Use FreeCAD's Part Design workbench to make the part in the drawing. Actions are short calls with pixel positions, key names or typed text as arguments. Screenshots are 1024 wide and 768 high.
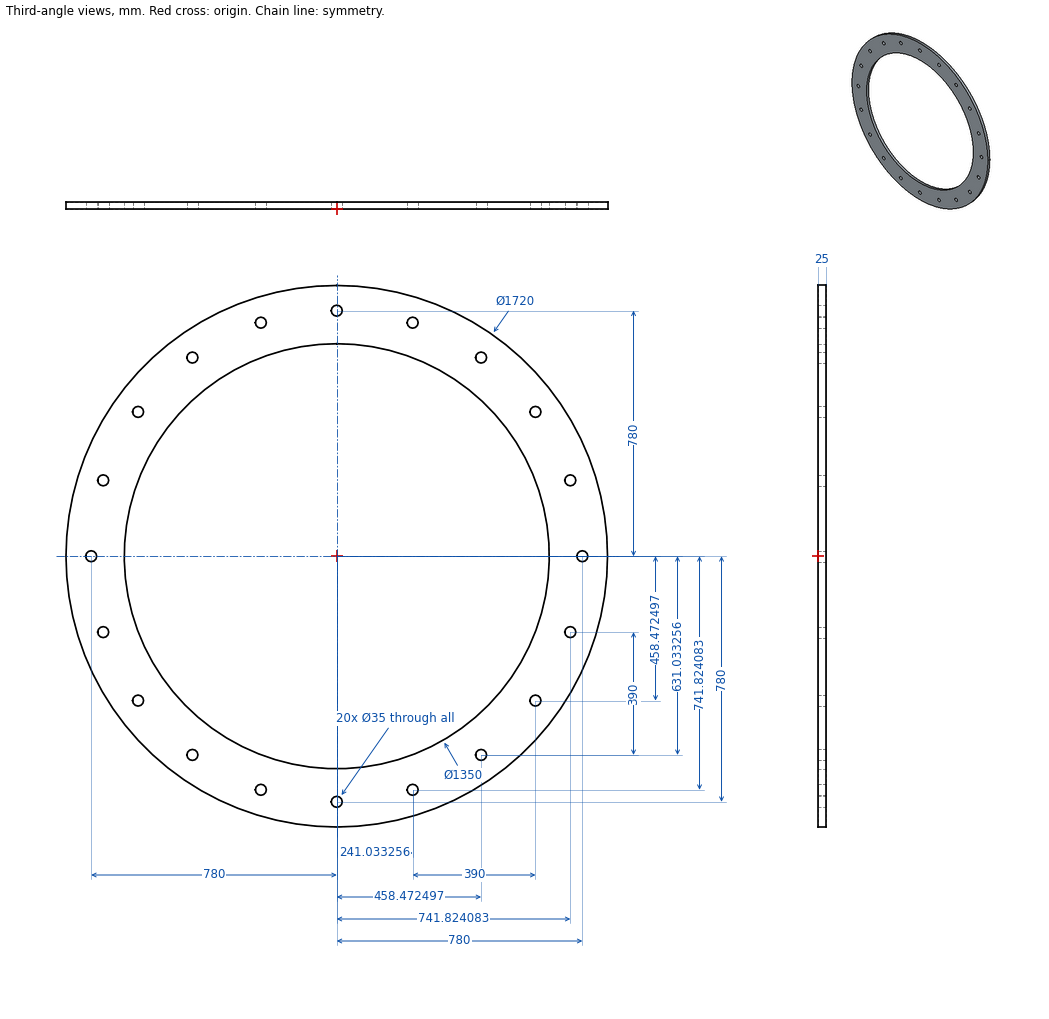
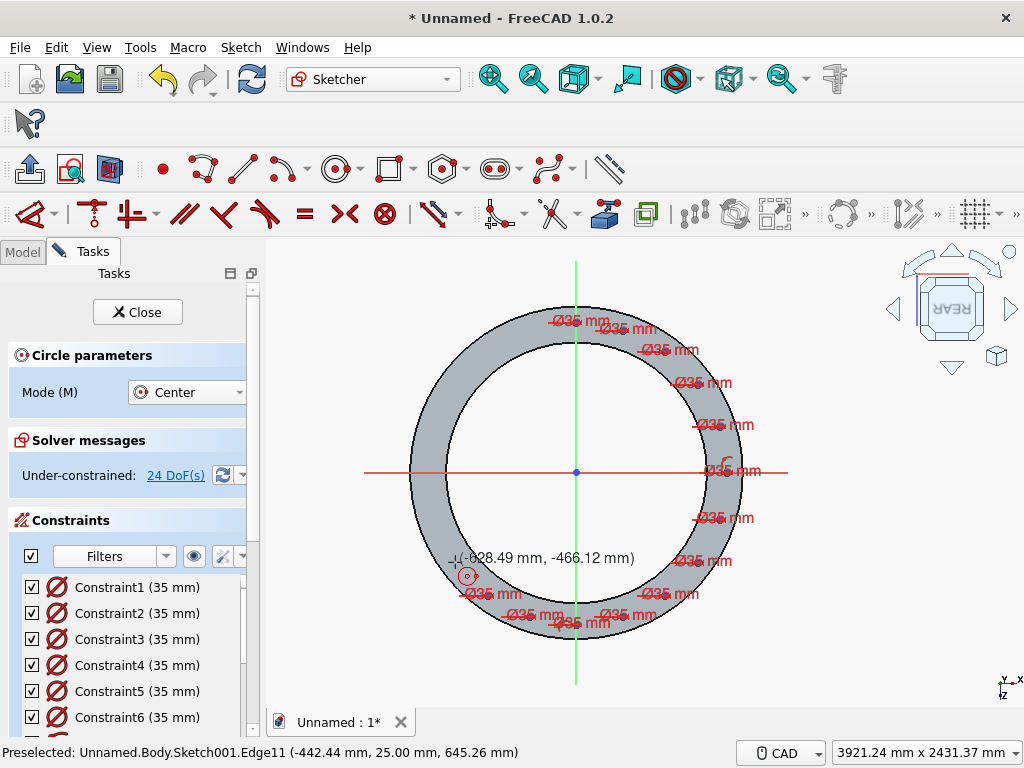
click(455, 562)
move(457, 559)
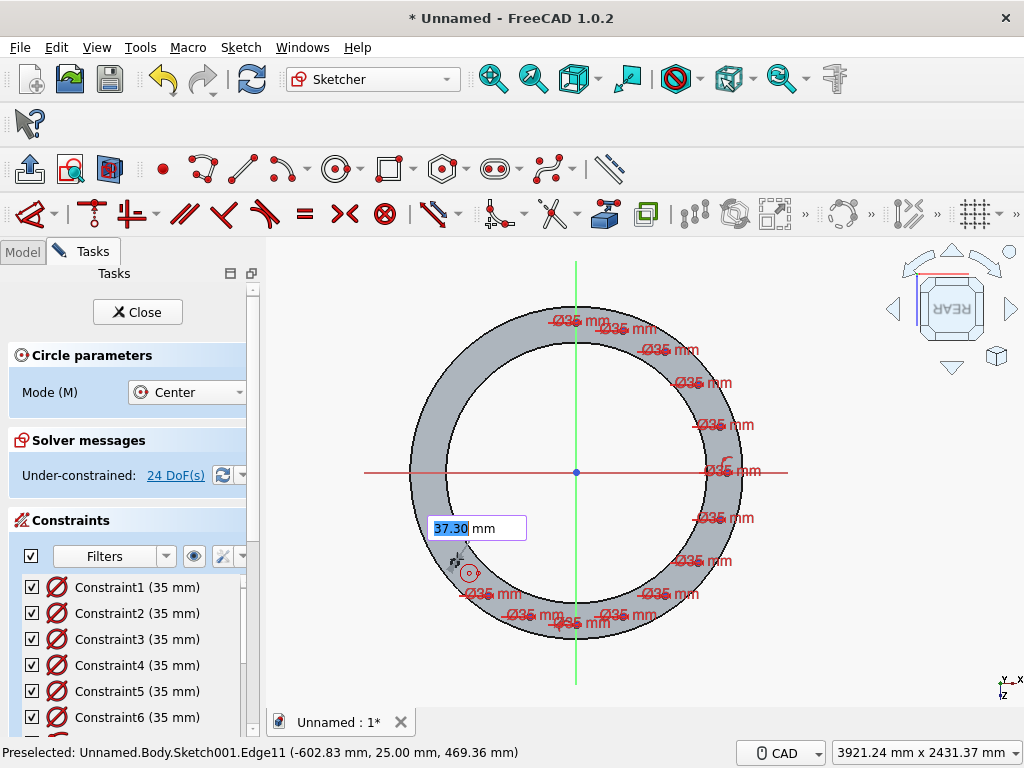
text(35)
key(Return)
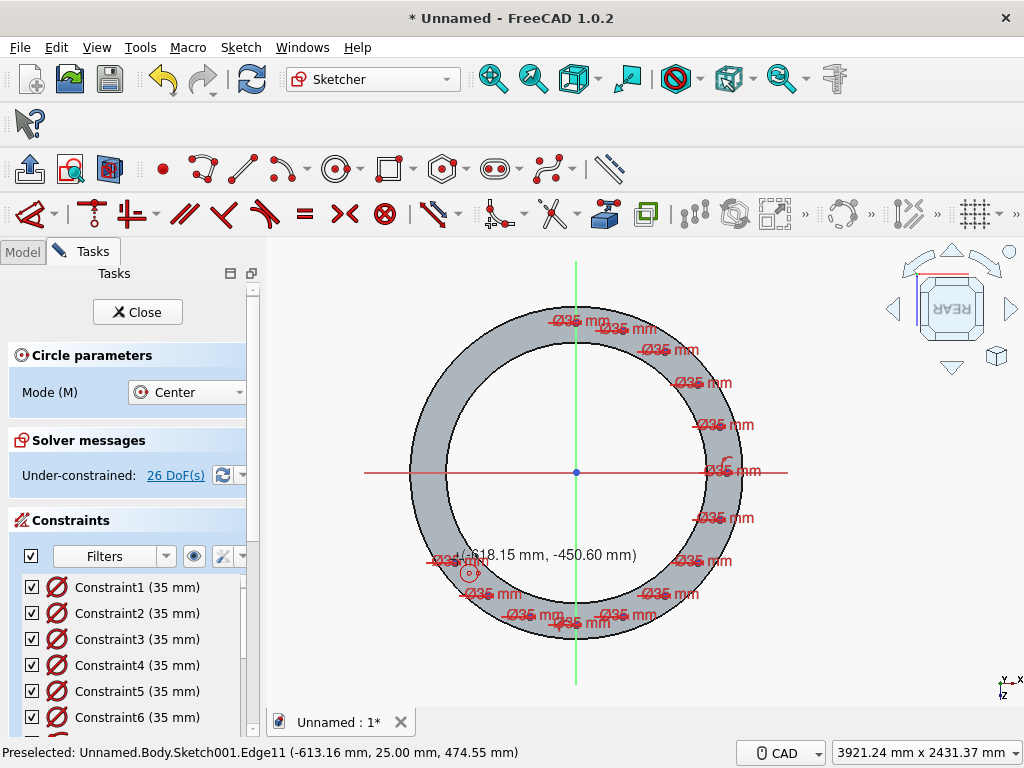
scroll(433, 519, up, 10)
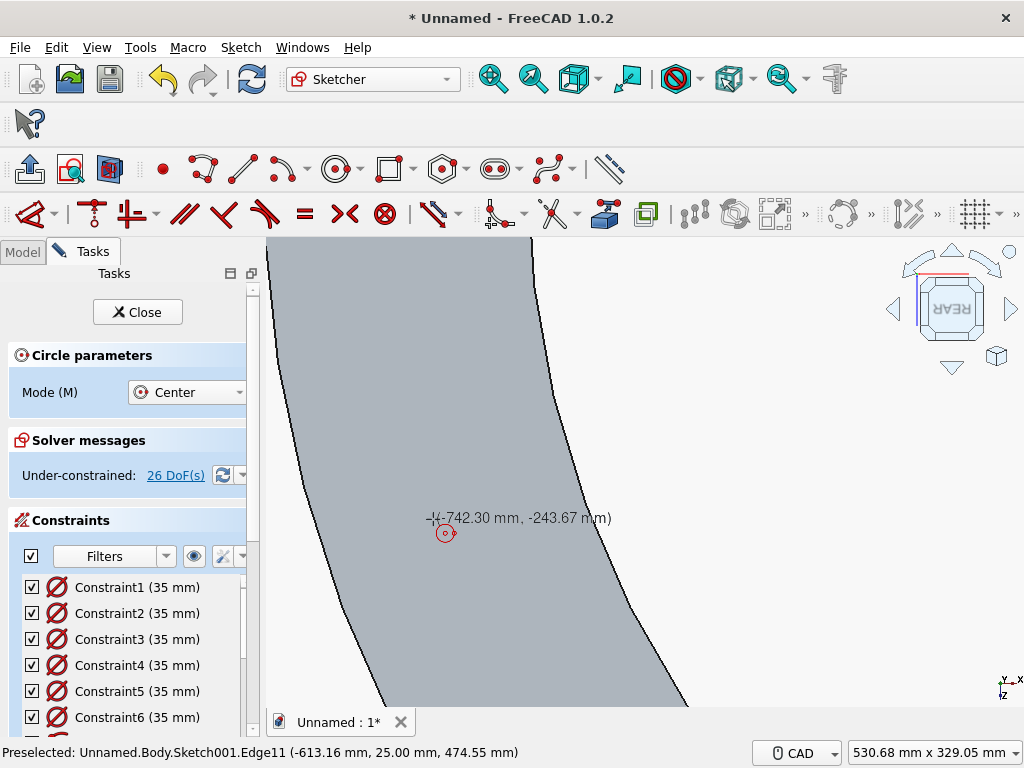
scroll(433, 519, down, 10)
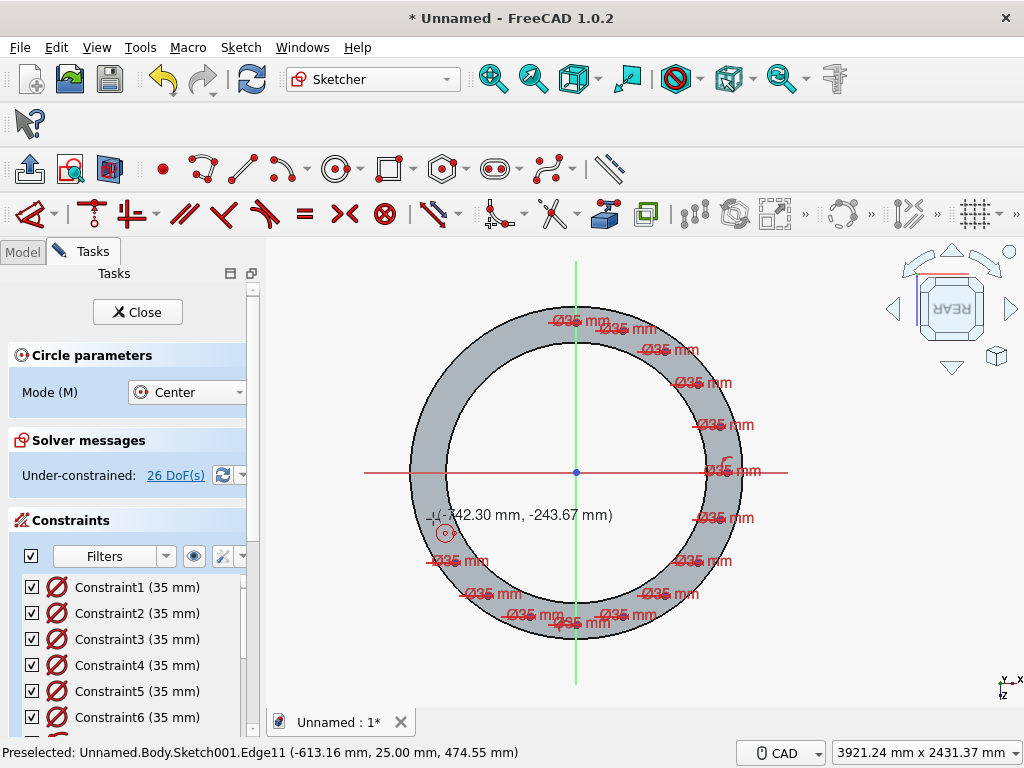
click(433, 519)
move(435, 517)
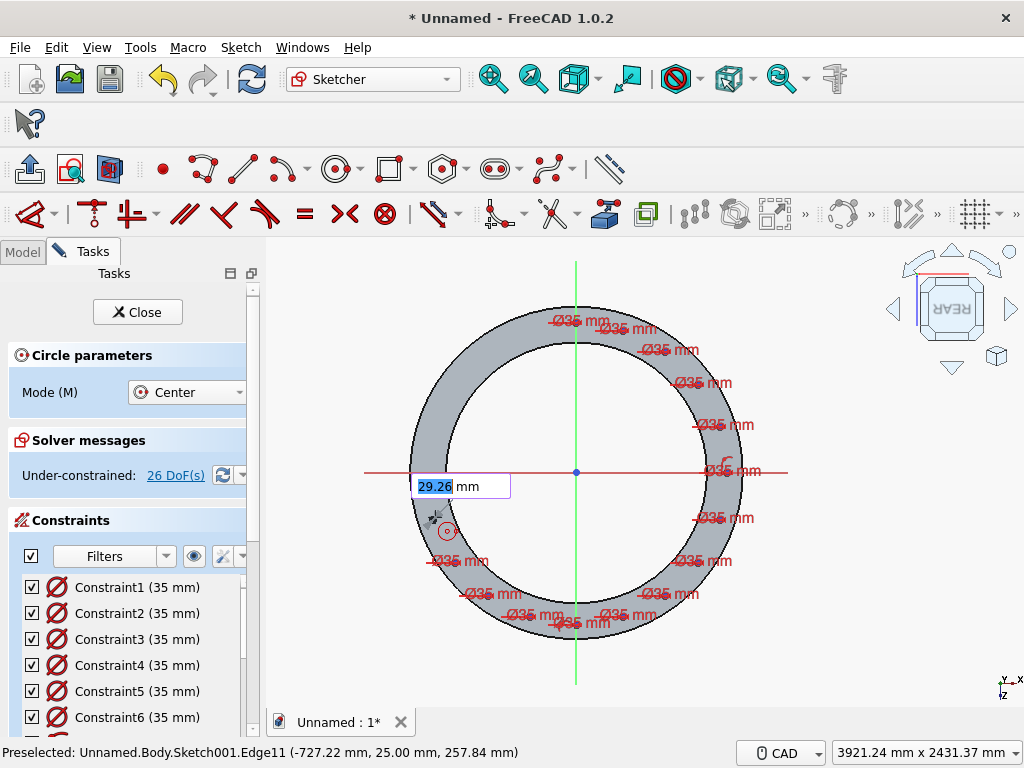
text(35)
key(Return)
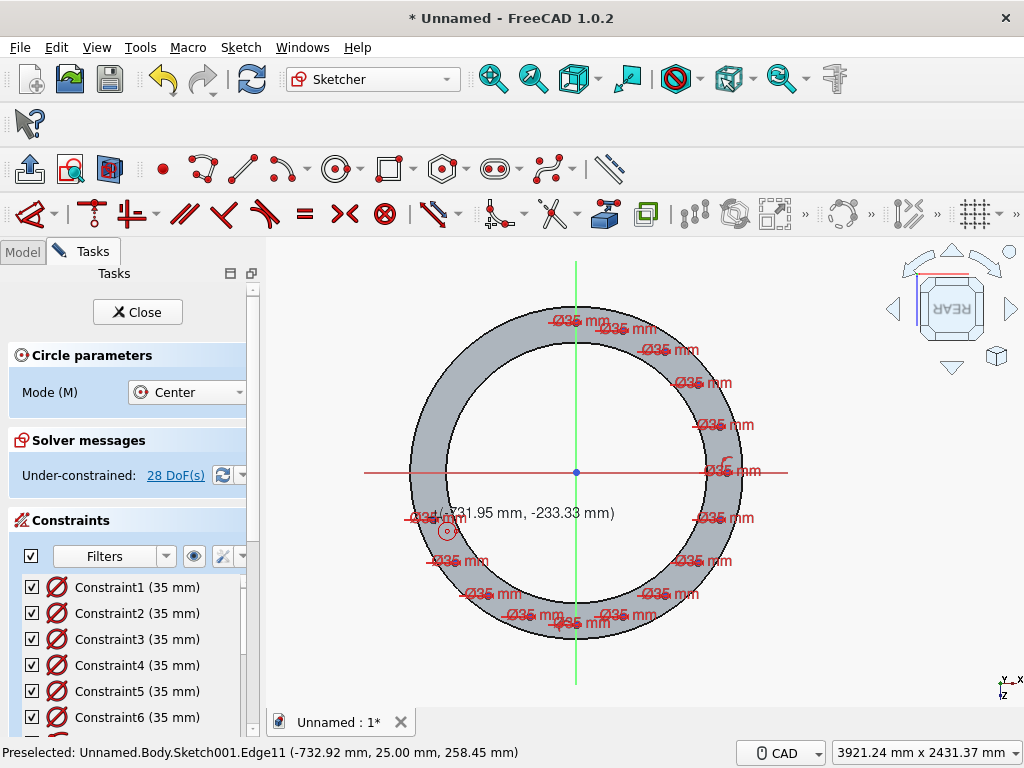
scroll(426, 473, up, 10)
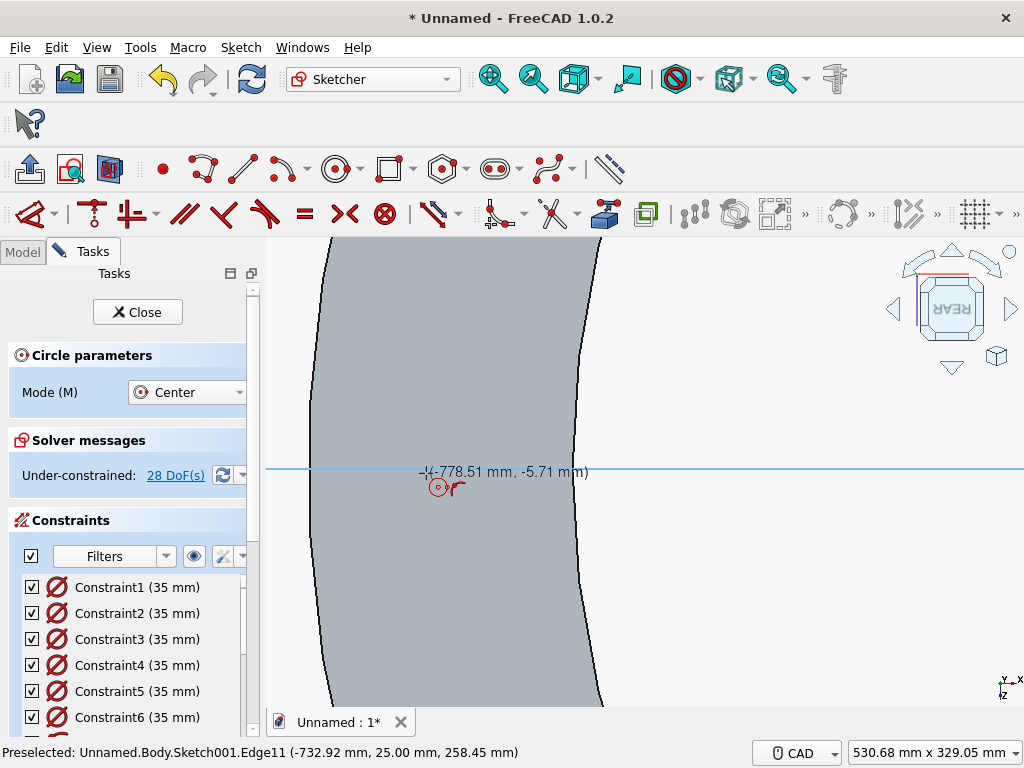
scroll(426, 472, down, 10)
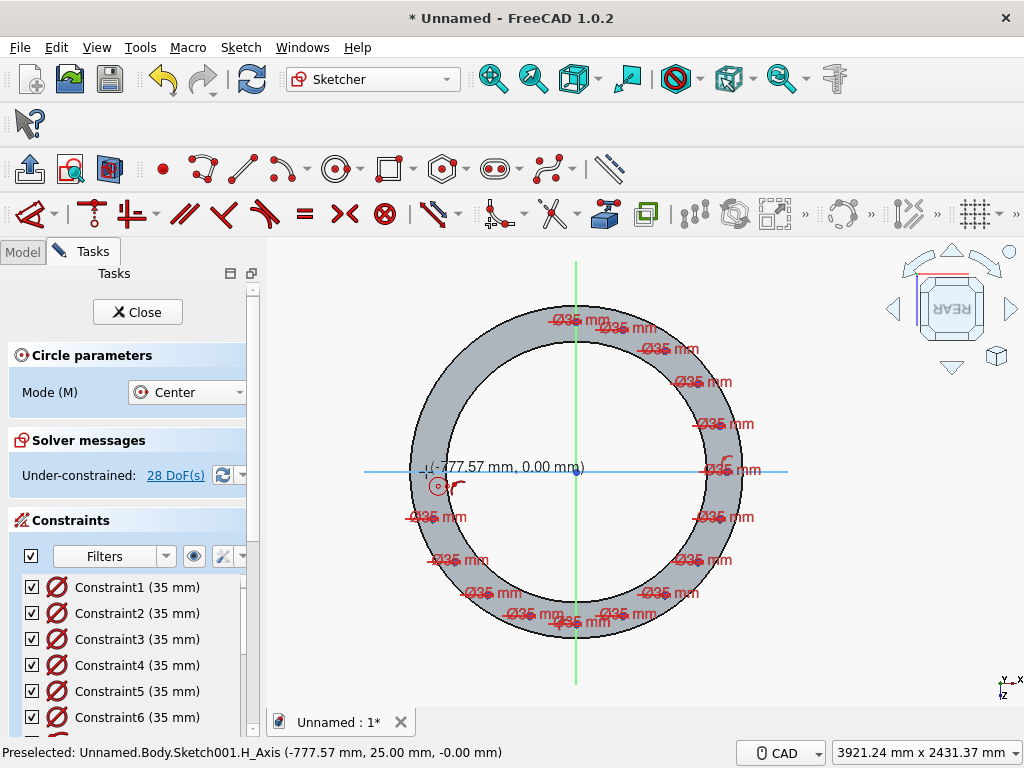
click(426, 472)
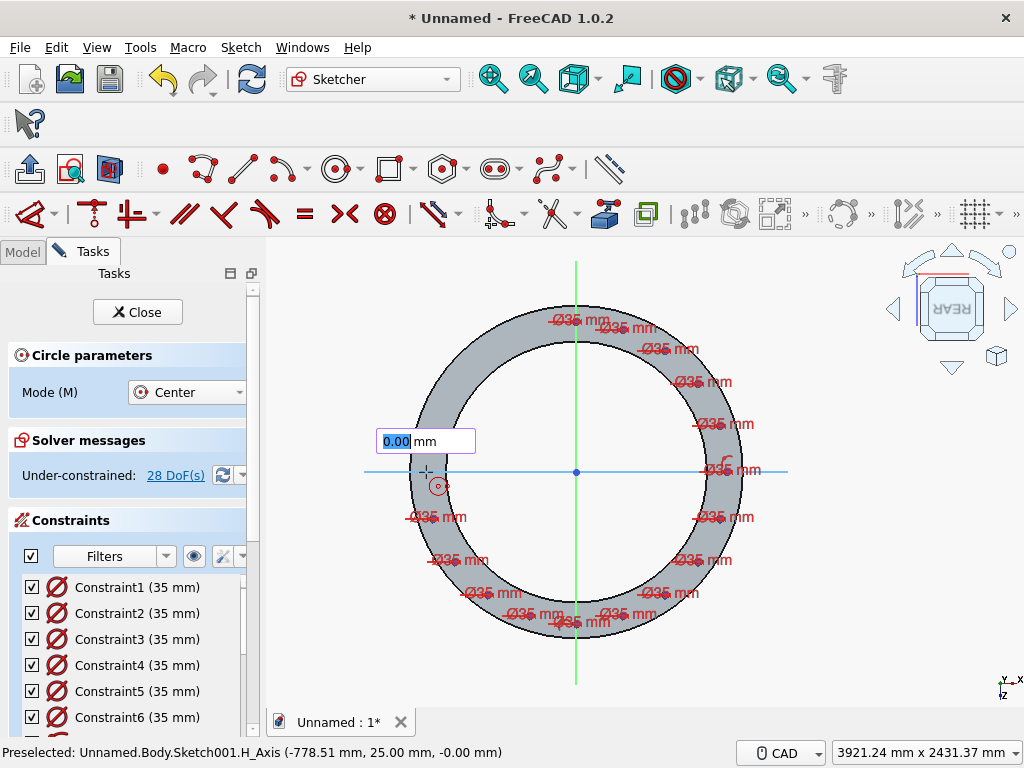
scroll(427, 469, up, 9)
move(425, 466)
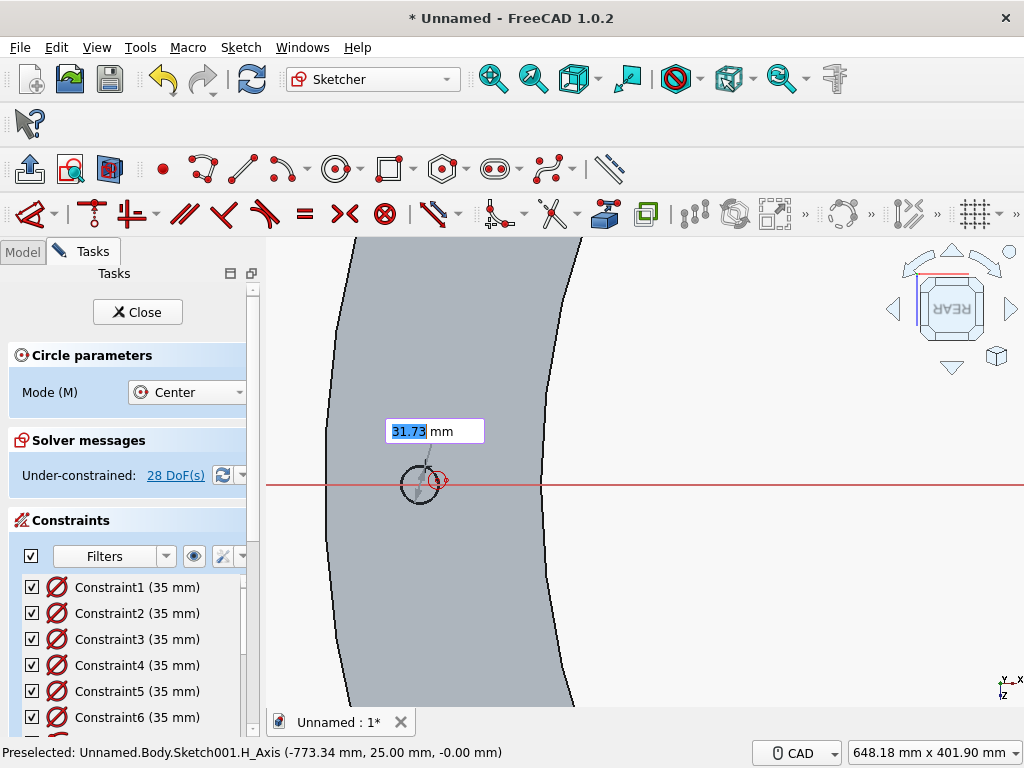
text(35)
key(Return)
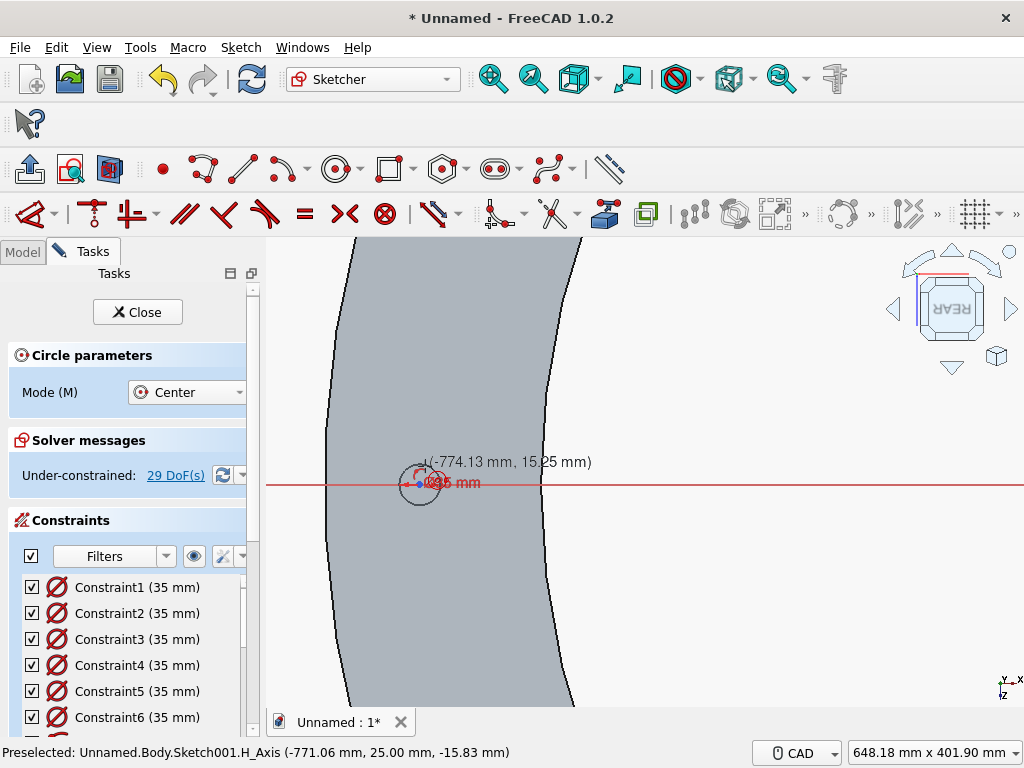
scroll(427, 469, down, 9)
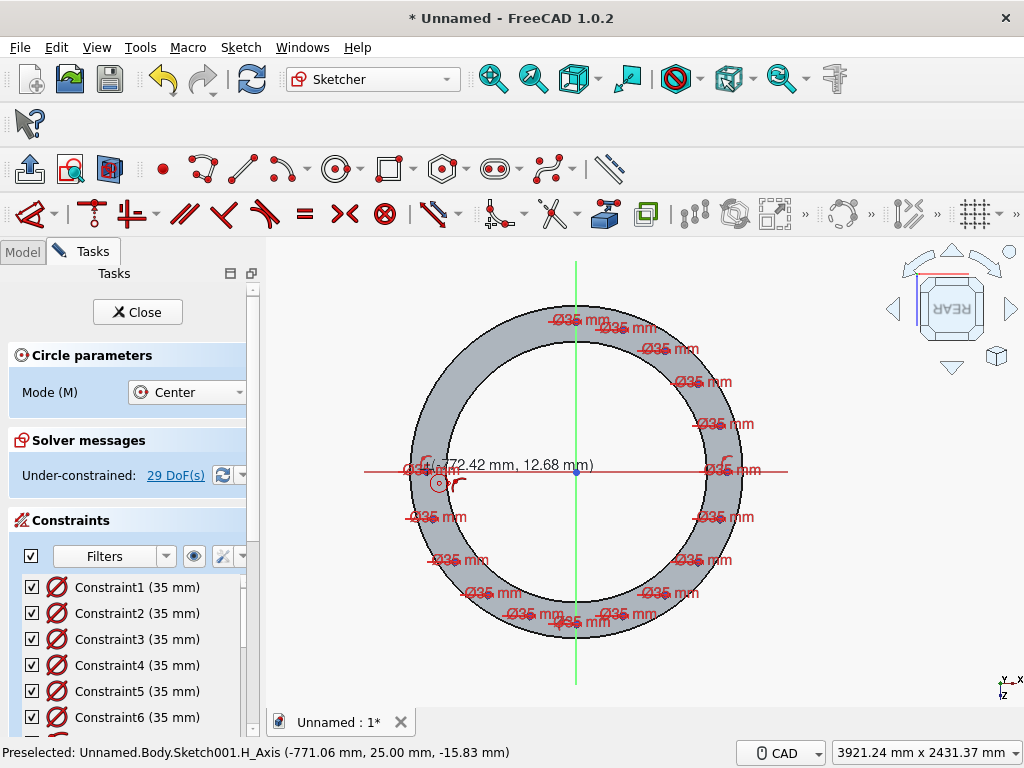
scroll(433, 425, up, 10)